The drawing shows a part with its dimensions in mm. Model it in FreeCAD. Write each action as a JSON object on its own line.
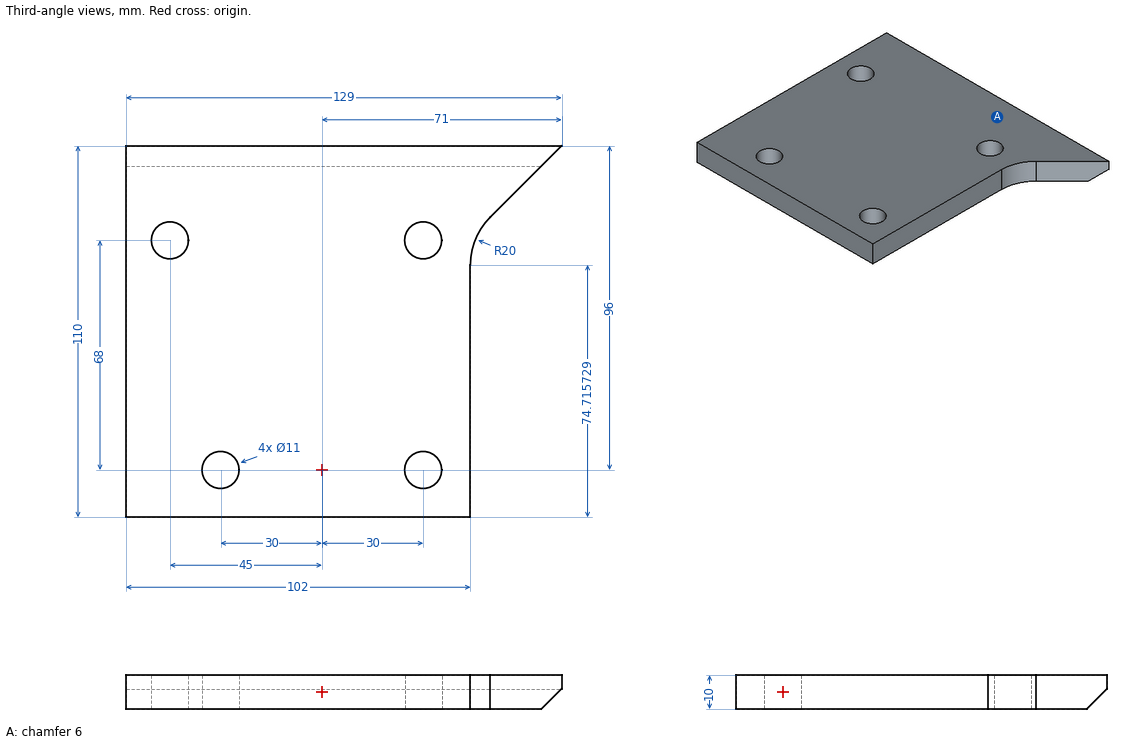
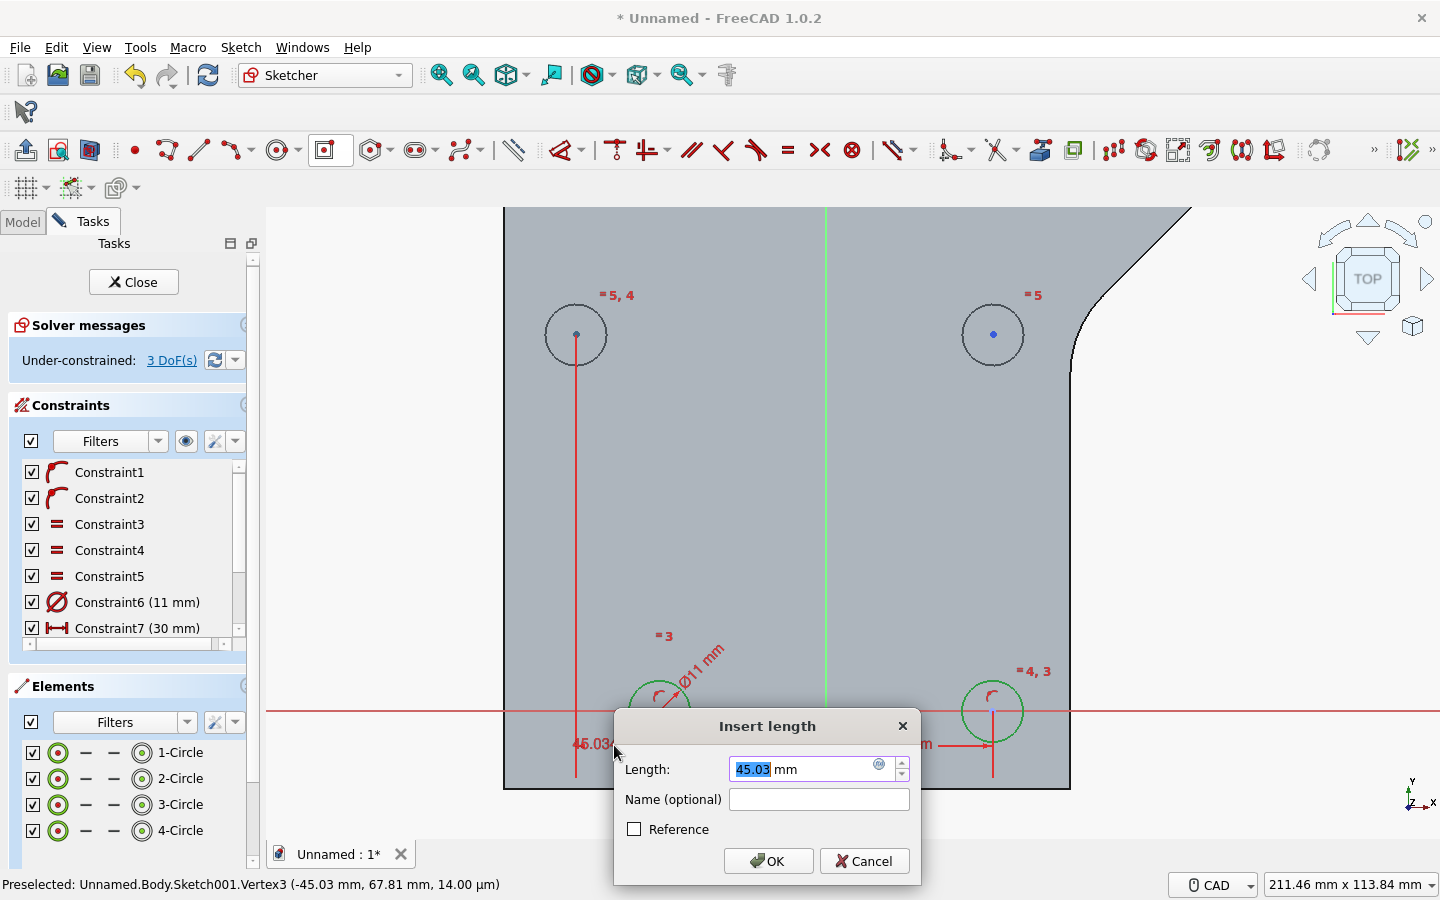
{"action": "type", "text": "45"}
{"action": "key", "text": "Return"}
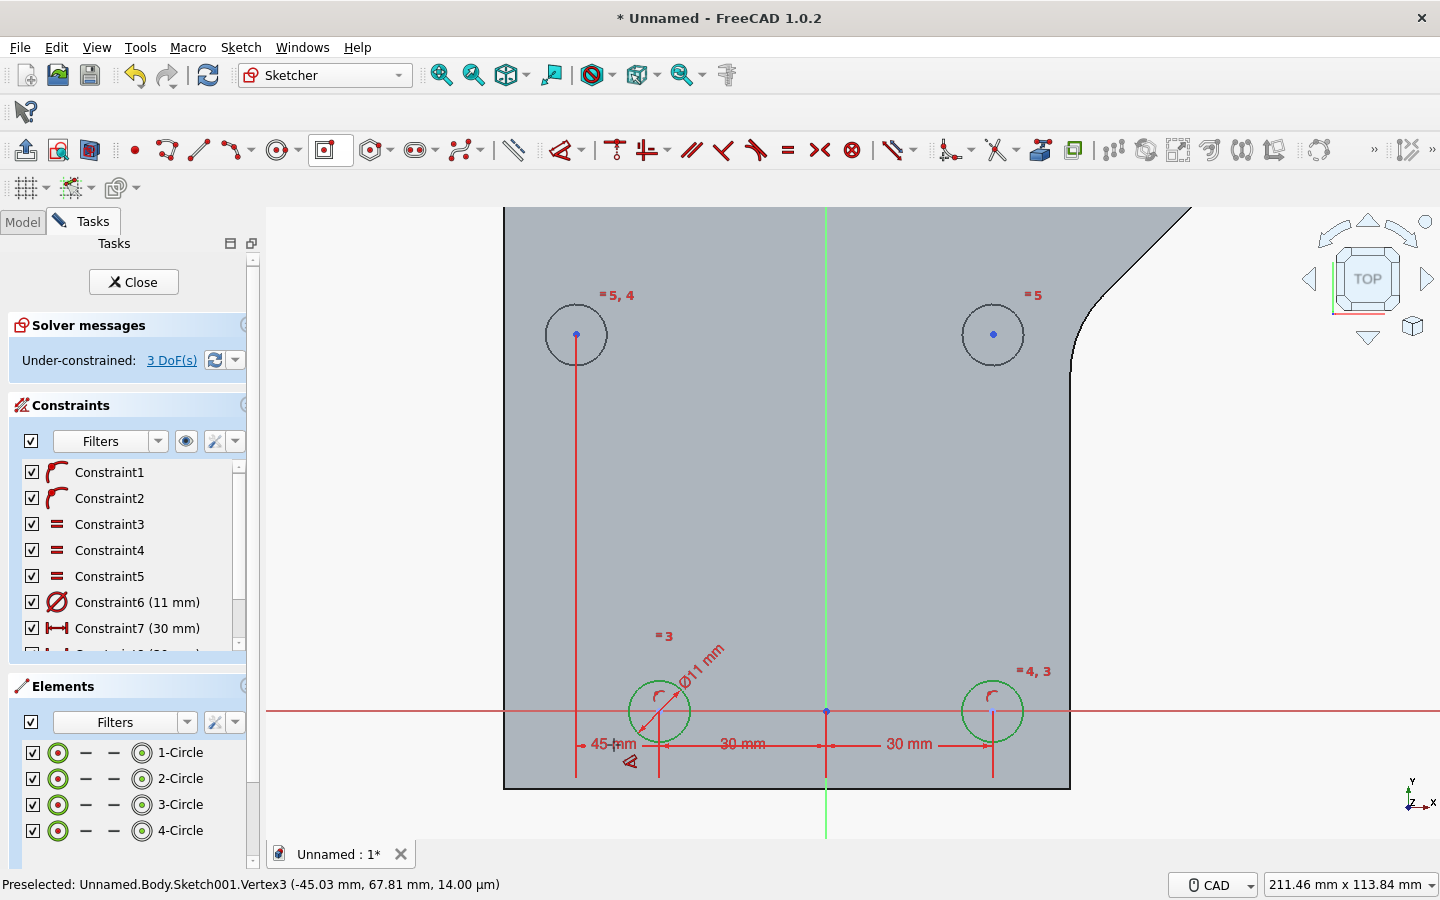
{"action": "left_click", "coordinate": [576, 335]}
{"action": "left_click", "coordinate": [542, 523]}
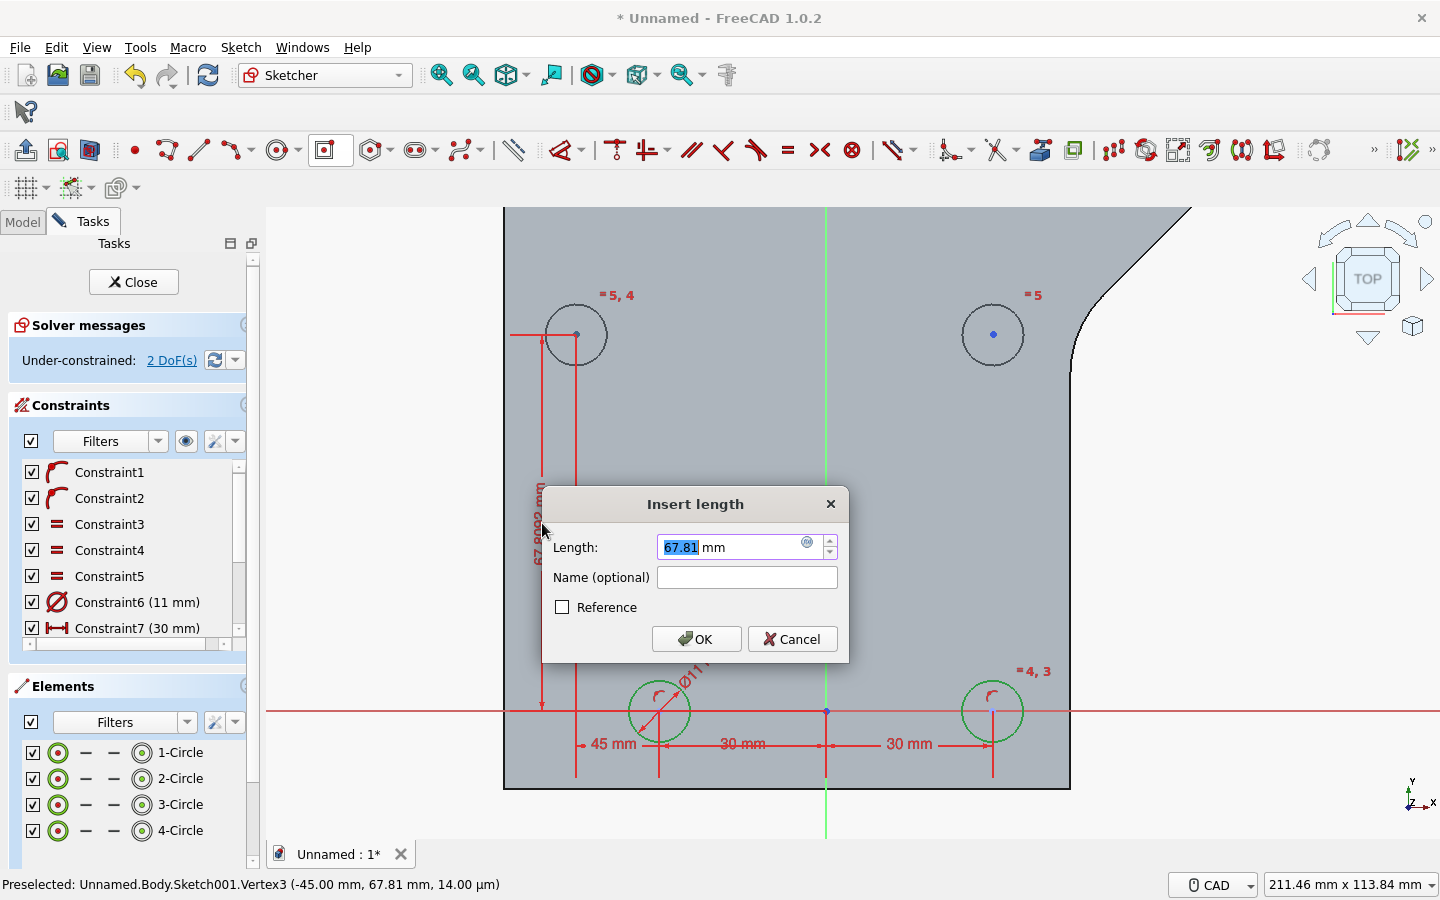
{"action": "type", "text": "68"}
{"action": "key", "text": "Return"}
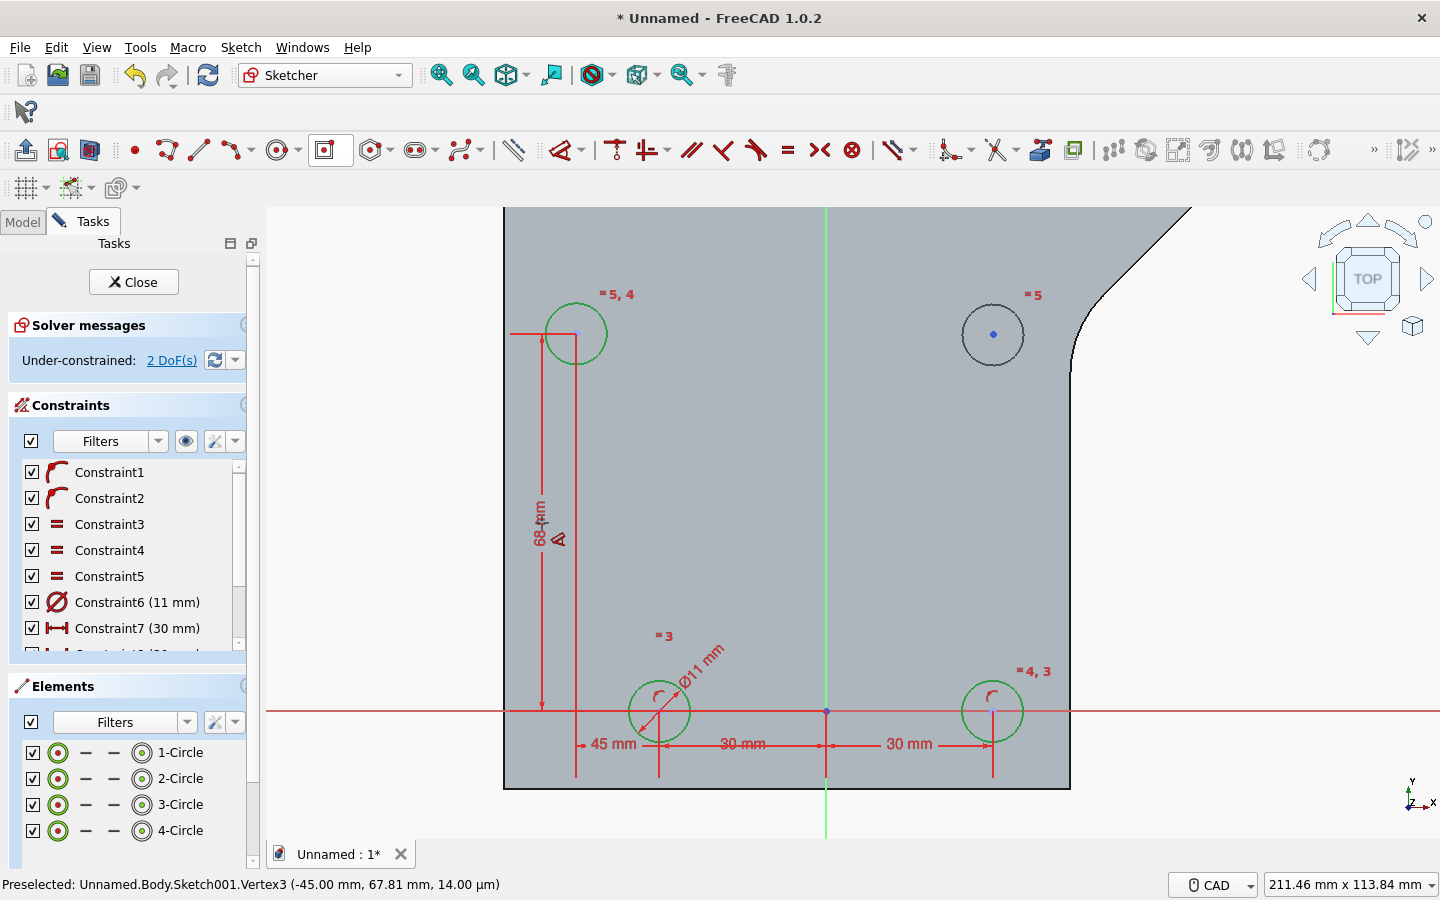
{"action": "left_click", "coordinate": [993, 335]}
{"action": "left_click", "coordinate": [910, 301]}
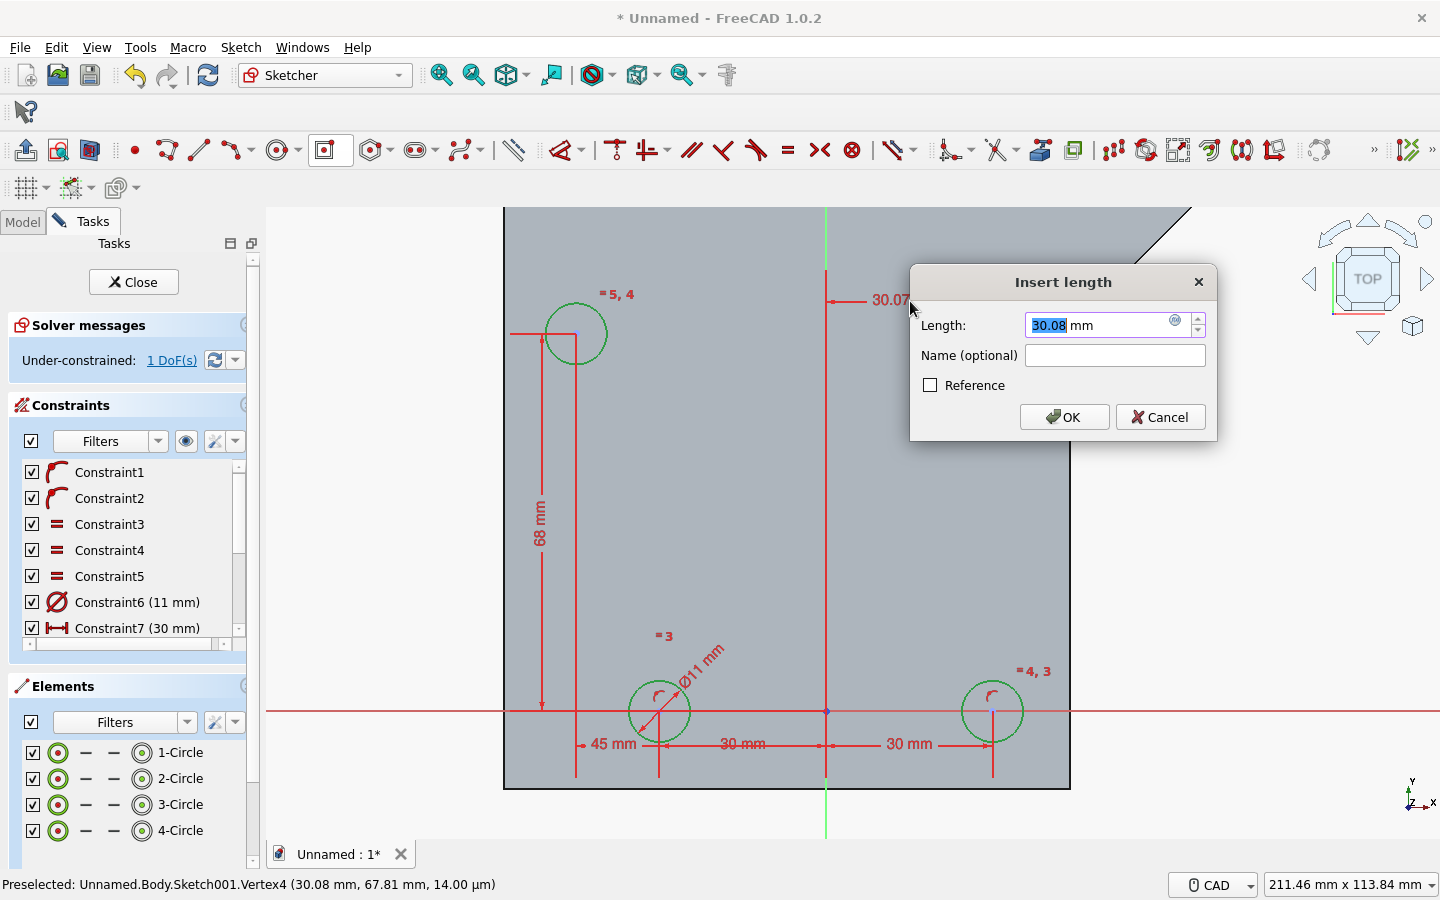
{"action": "type", "text": "30"}
{"action": "key", "text": "Return"}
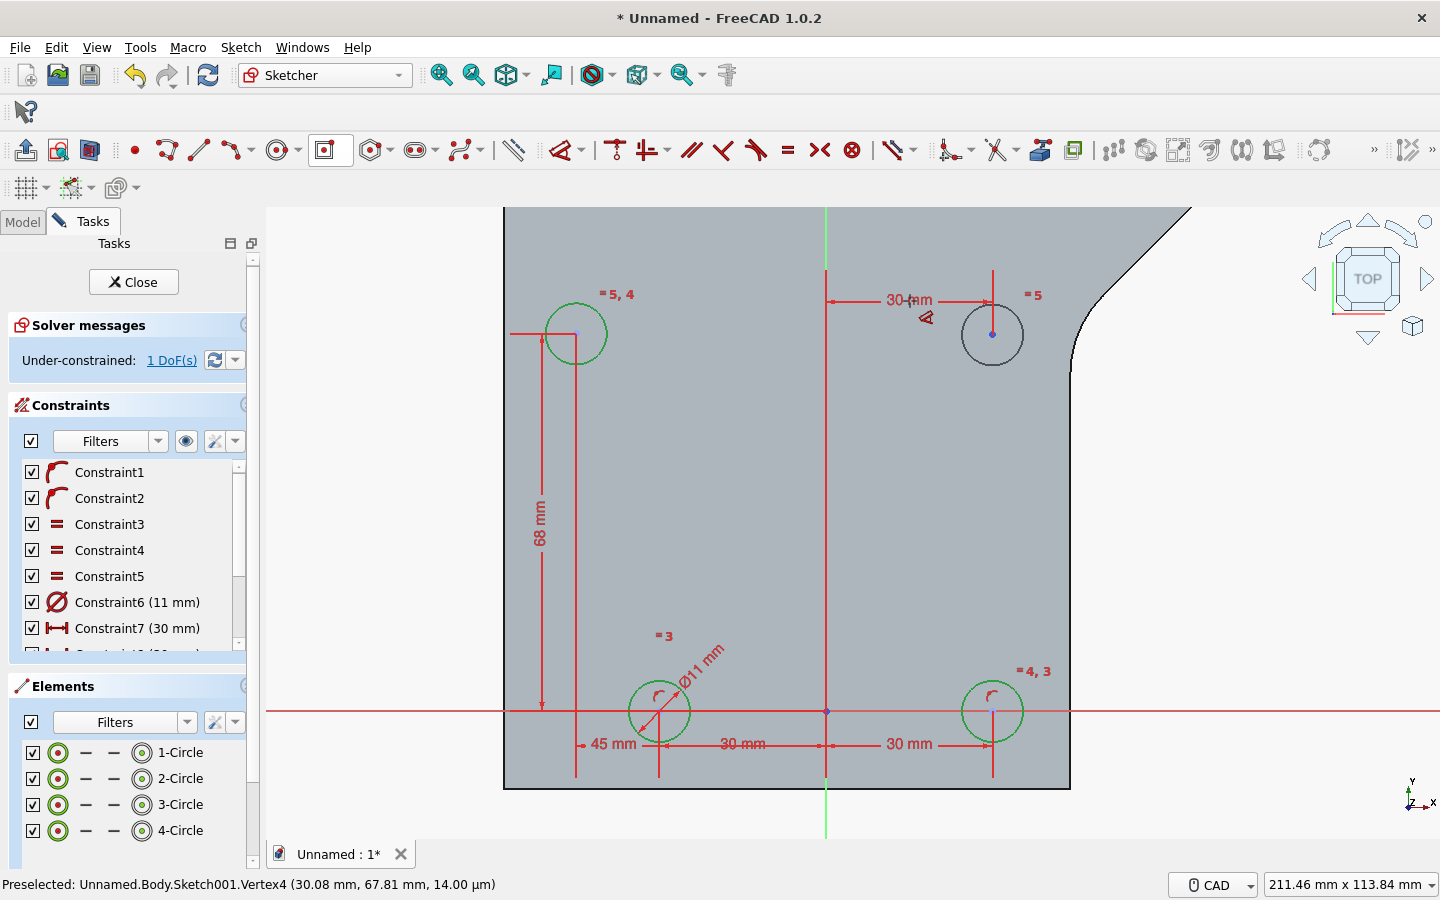
{"action": "left_click", "coordinate": [993, 335]}
{"action": "left_click", "coordinate": [1027, 523]}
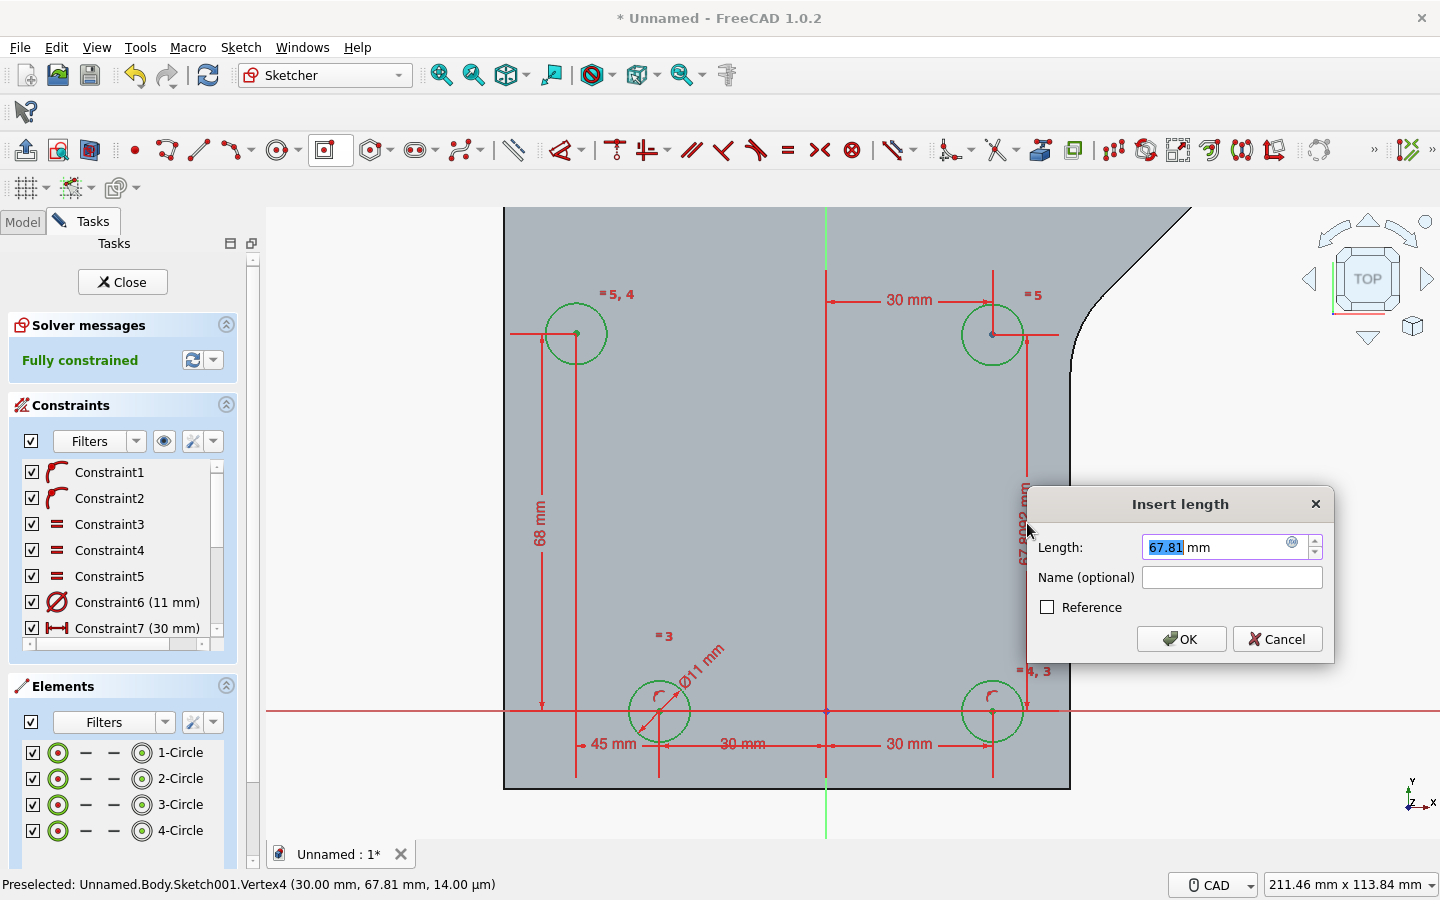
{"action": "type", "text": "68"}
{"action": "key", "text": "Return"}
{"action": "key", "text": "Escape"}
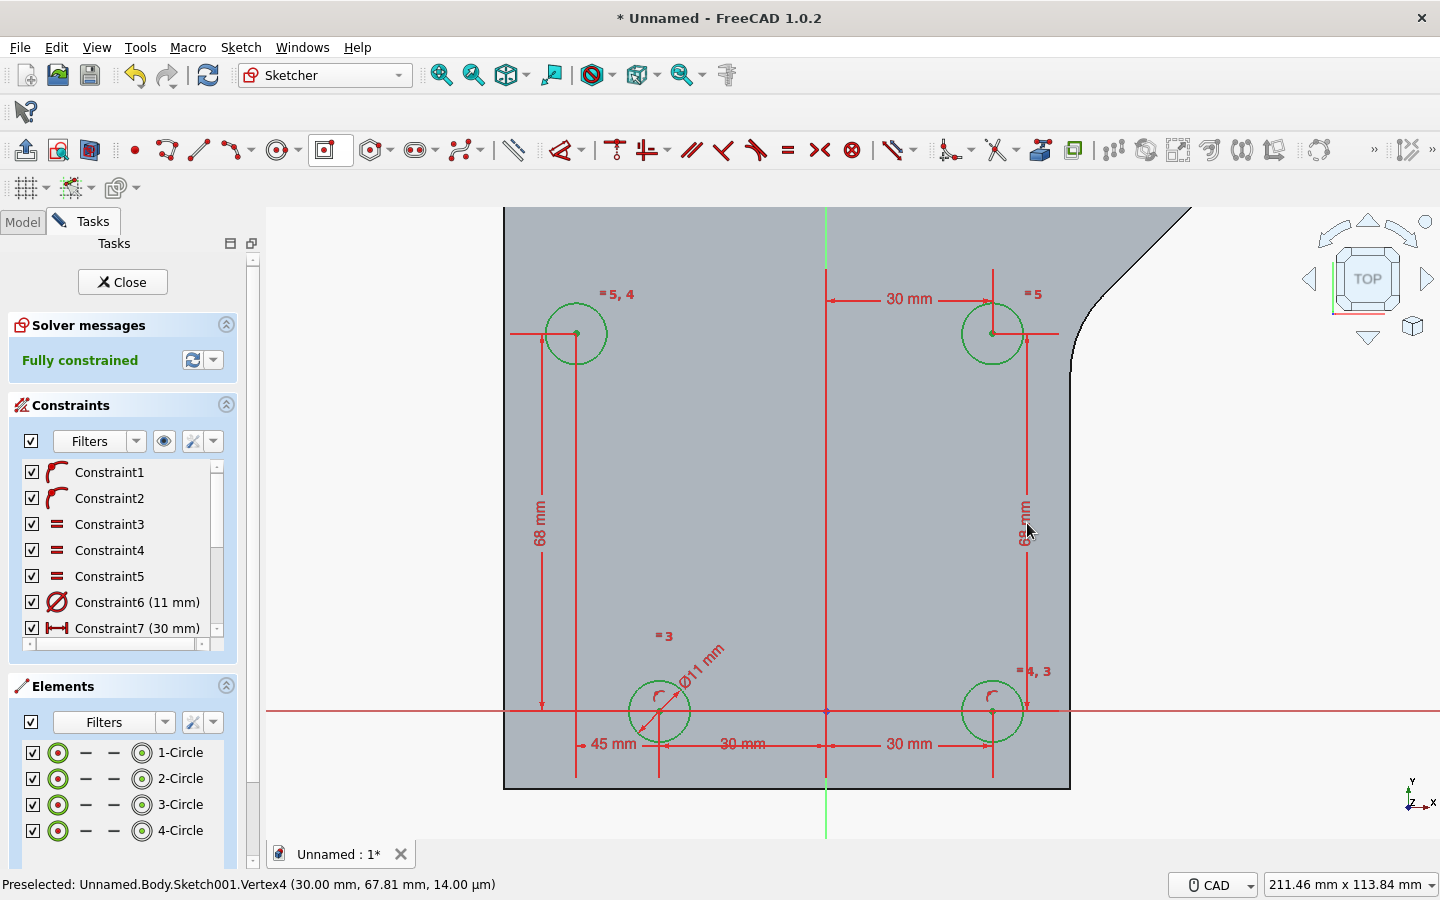
{"action": "left_click", "coordinate": [123, 282]}